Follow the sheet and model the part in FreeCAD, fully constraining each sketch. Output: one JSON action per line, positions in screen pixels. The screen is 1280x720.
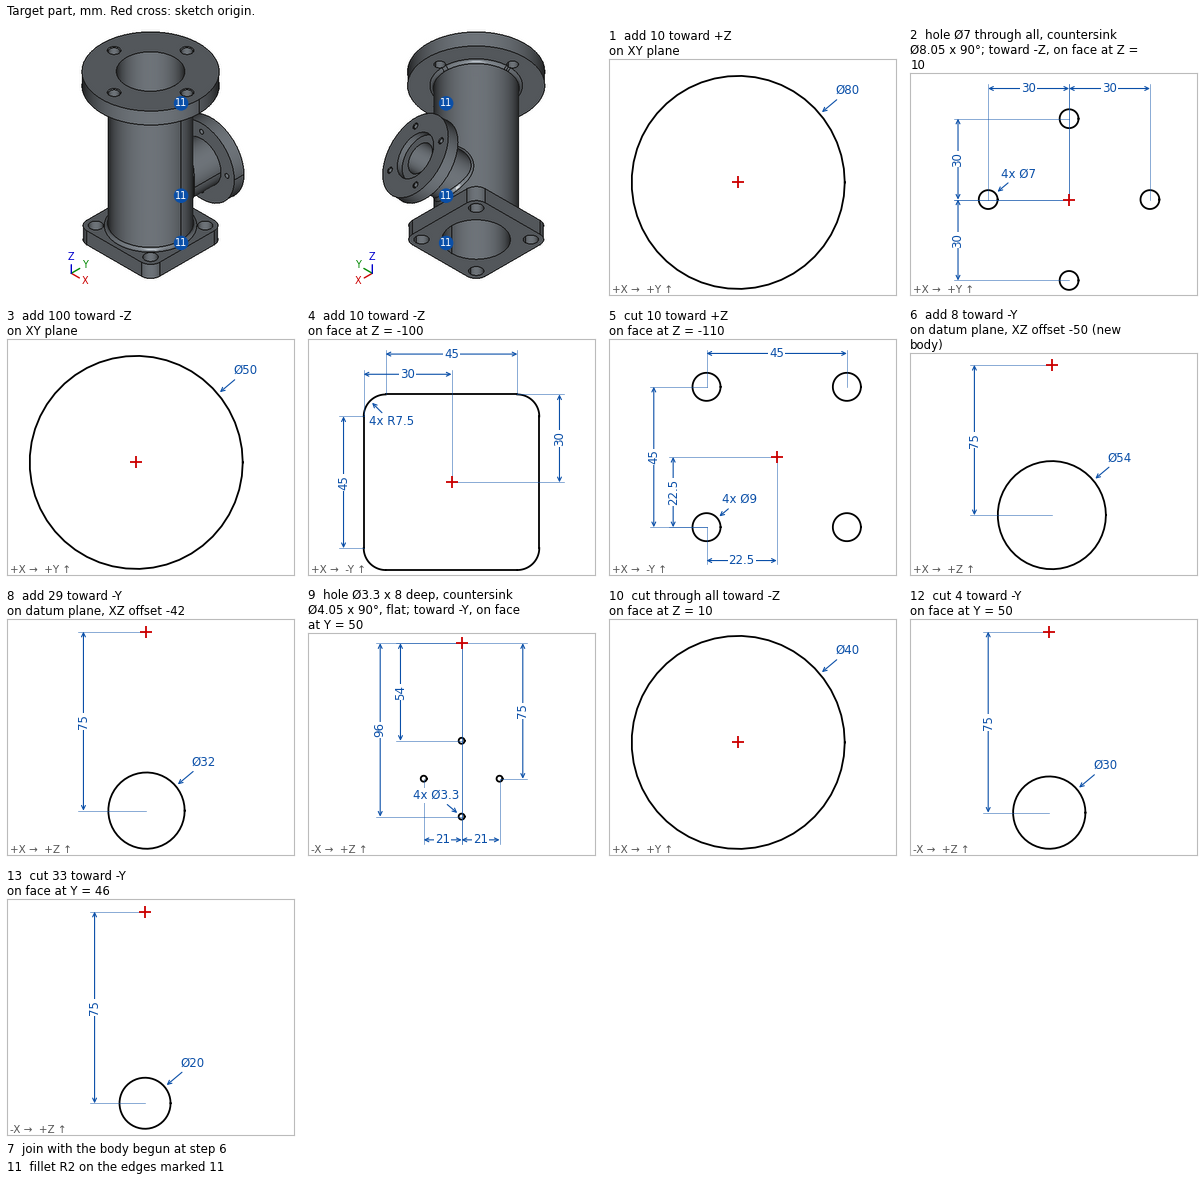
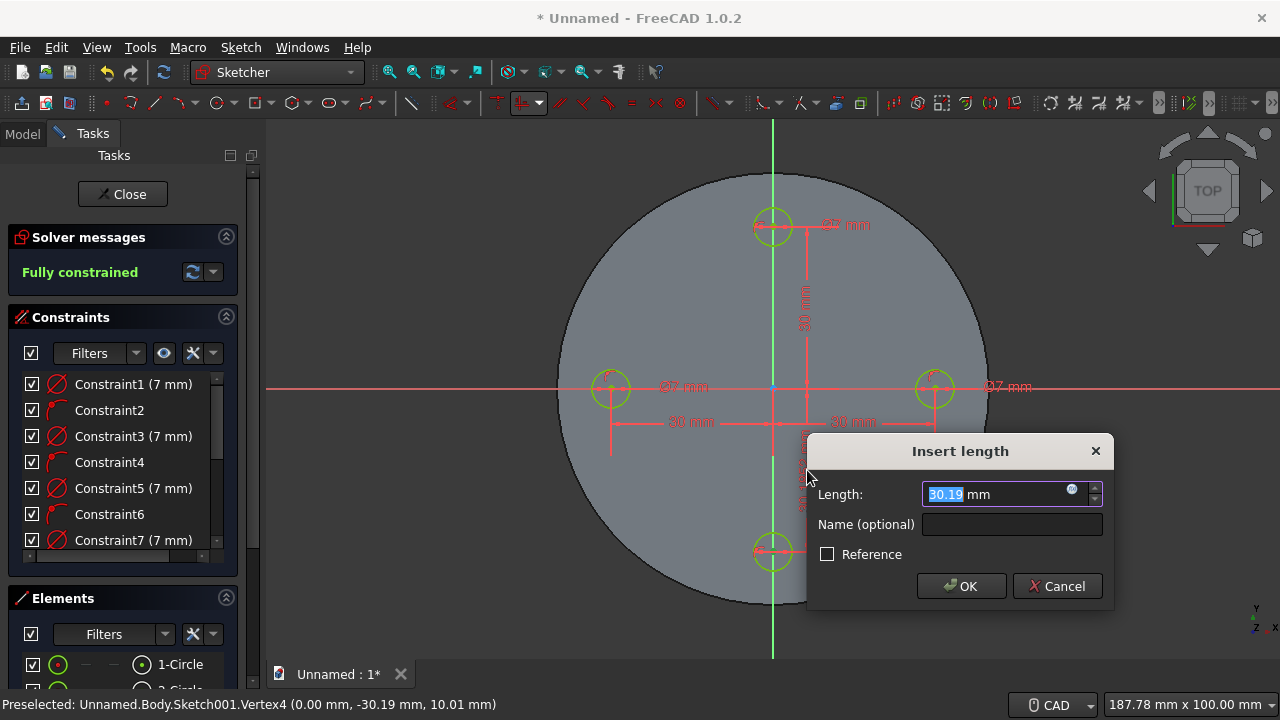
{"action": "type", "text": "30"}
{"action": "key", "text": "Return"}
{"action": "key", "text": "Escape"}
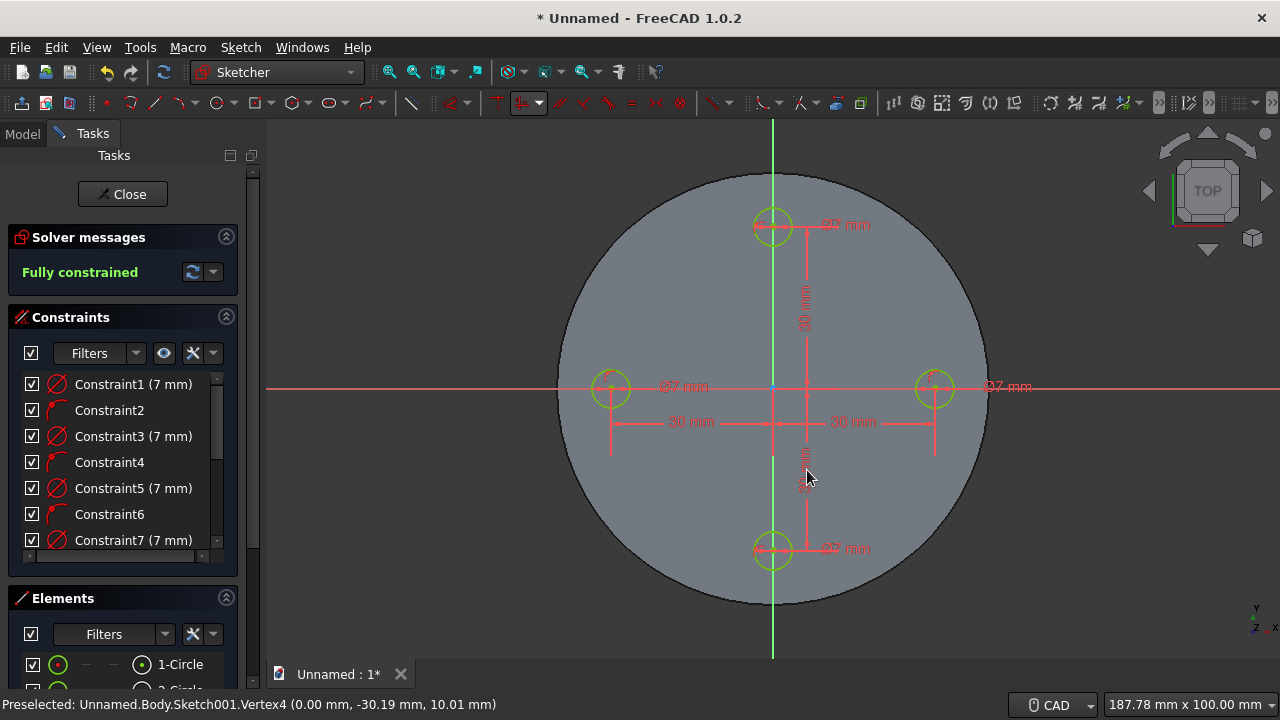
{"action": "left_click", "coordinate": [123, 194]}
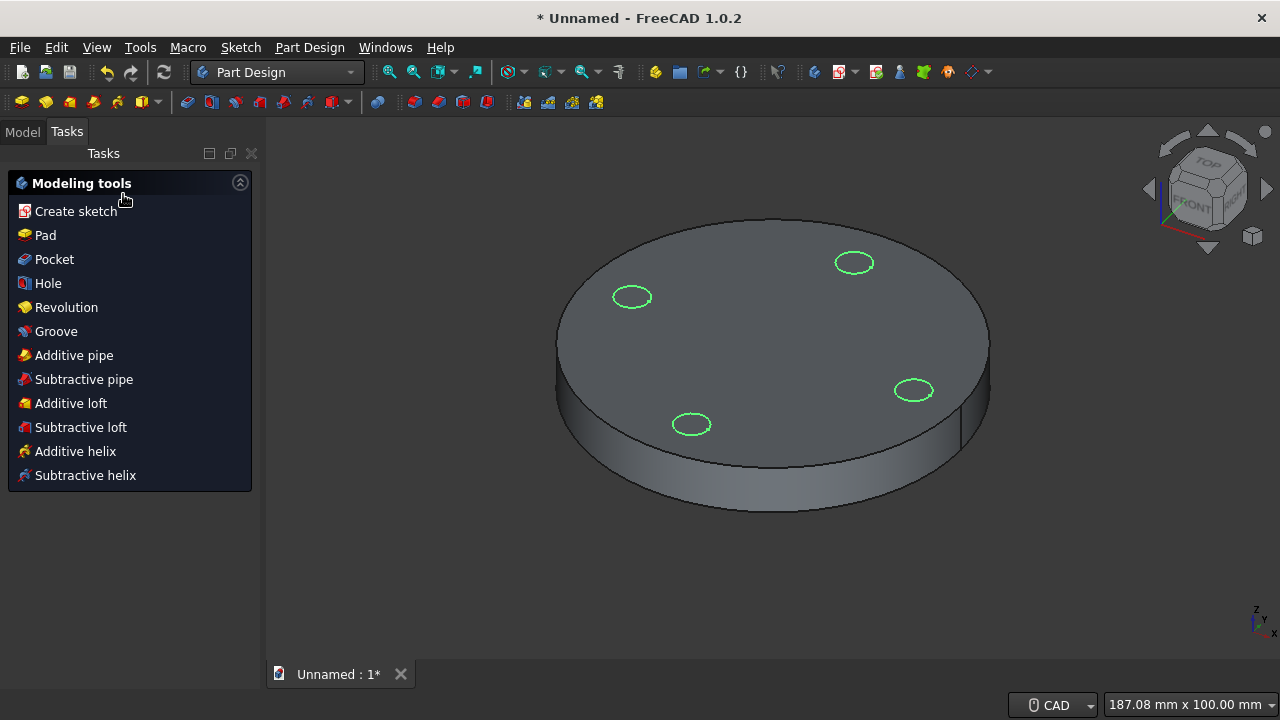
{"action": "left_click", "coordinate": [212, 102]}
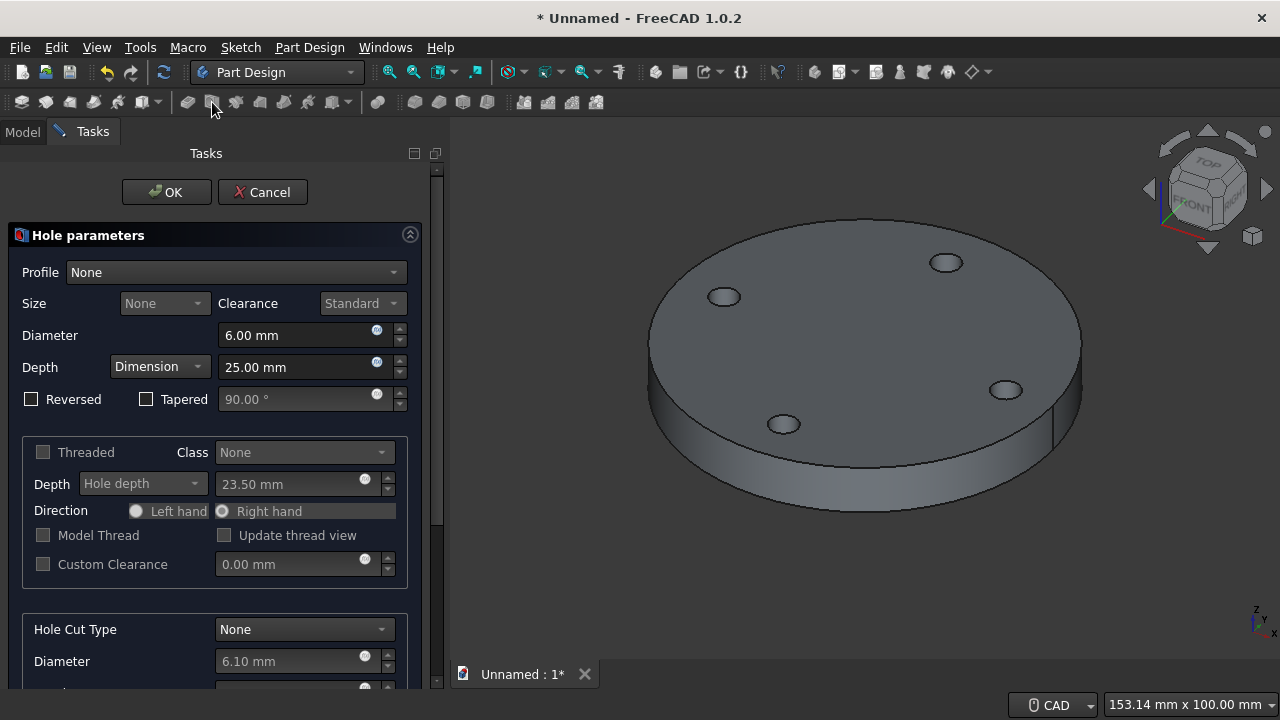
{"action": "triple_click", "coordinate": [305, 335]}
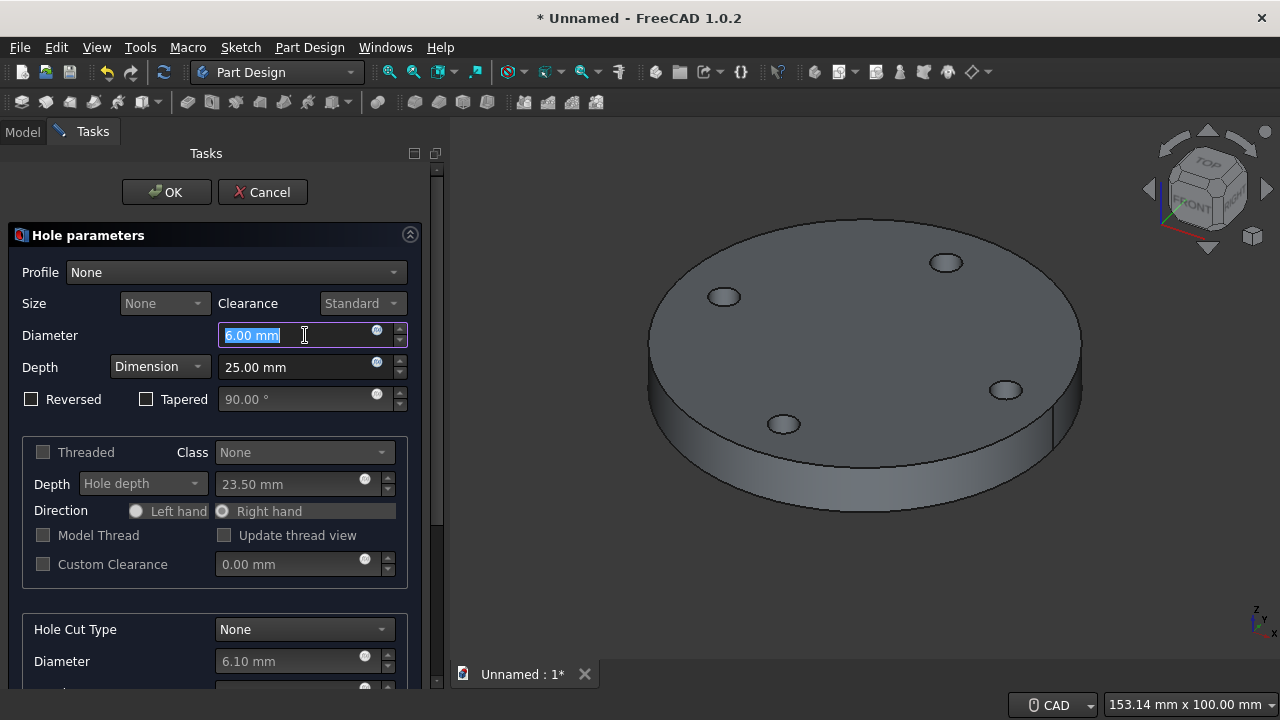
{"action": "type", "text": "7"}
{"action": "key", "text": "Tab"}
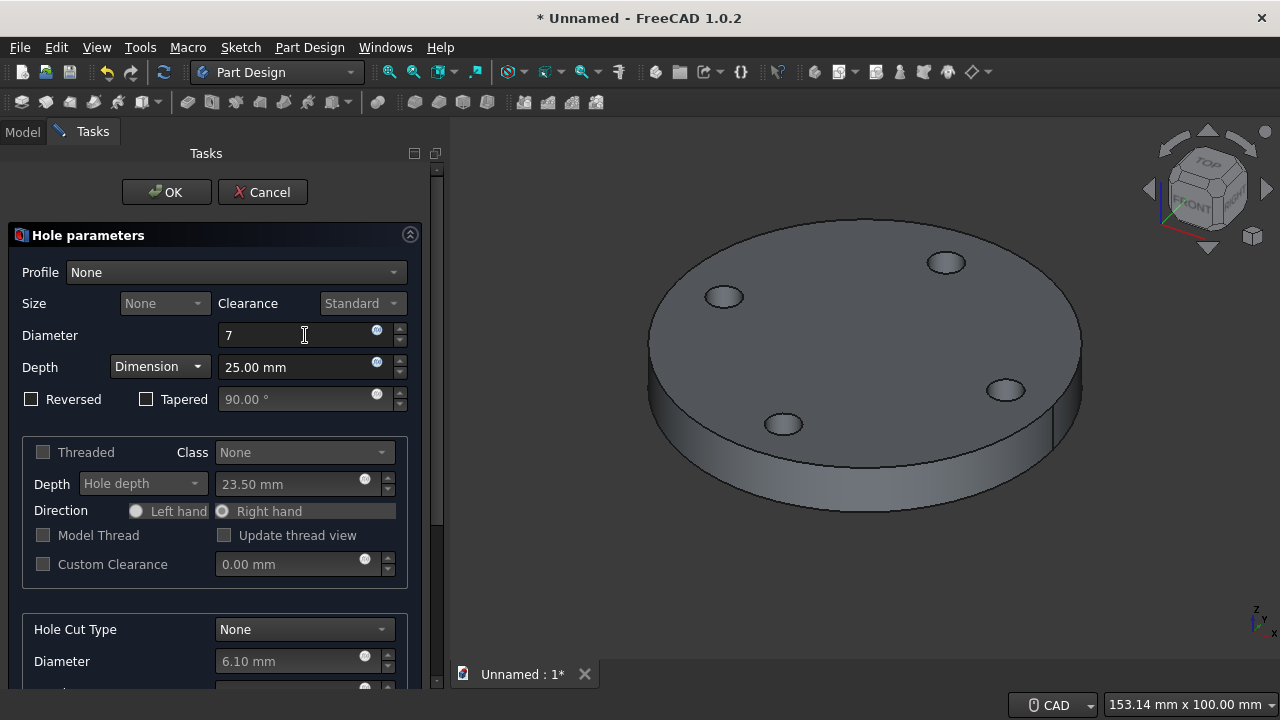
{"action": "left_click", "coordinate": [161, 366]}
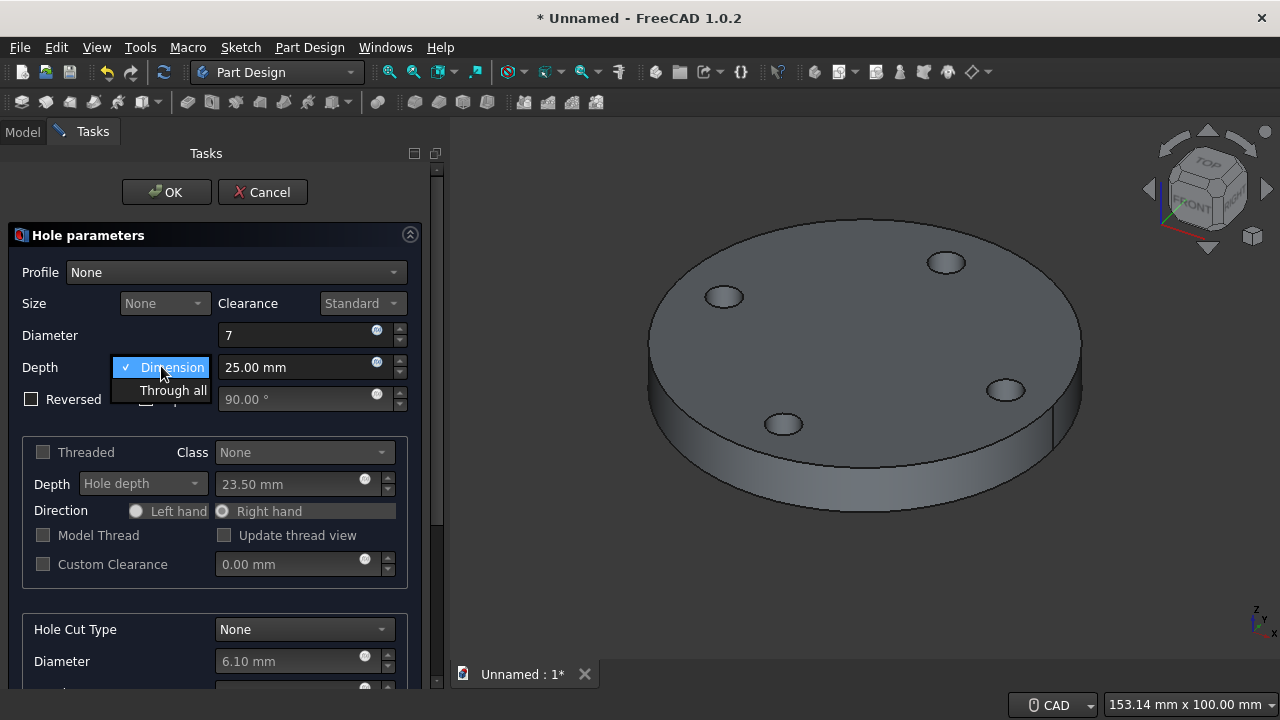
{"action": "left_click", "coordinate": [160, 390]}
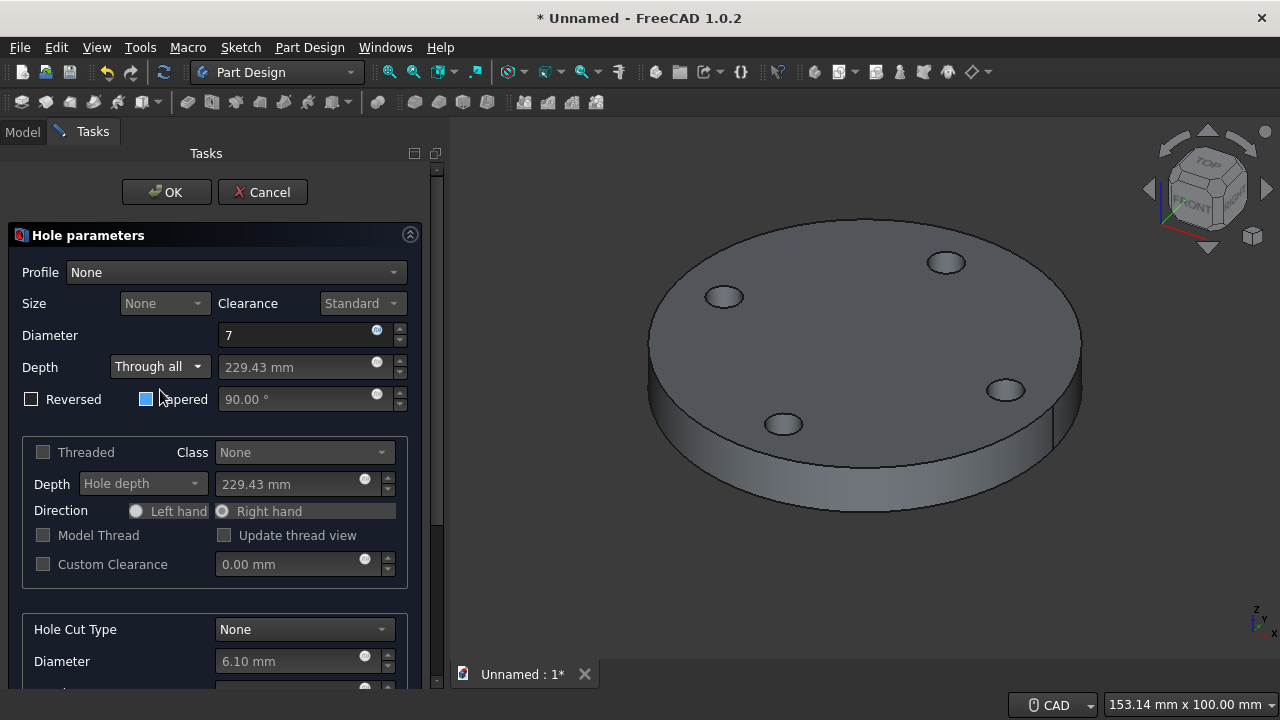
{"action": "left_click", "coordinate": [306, 630]}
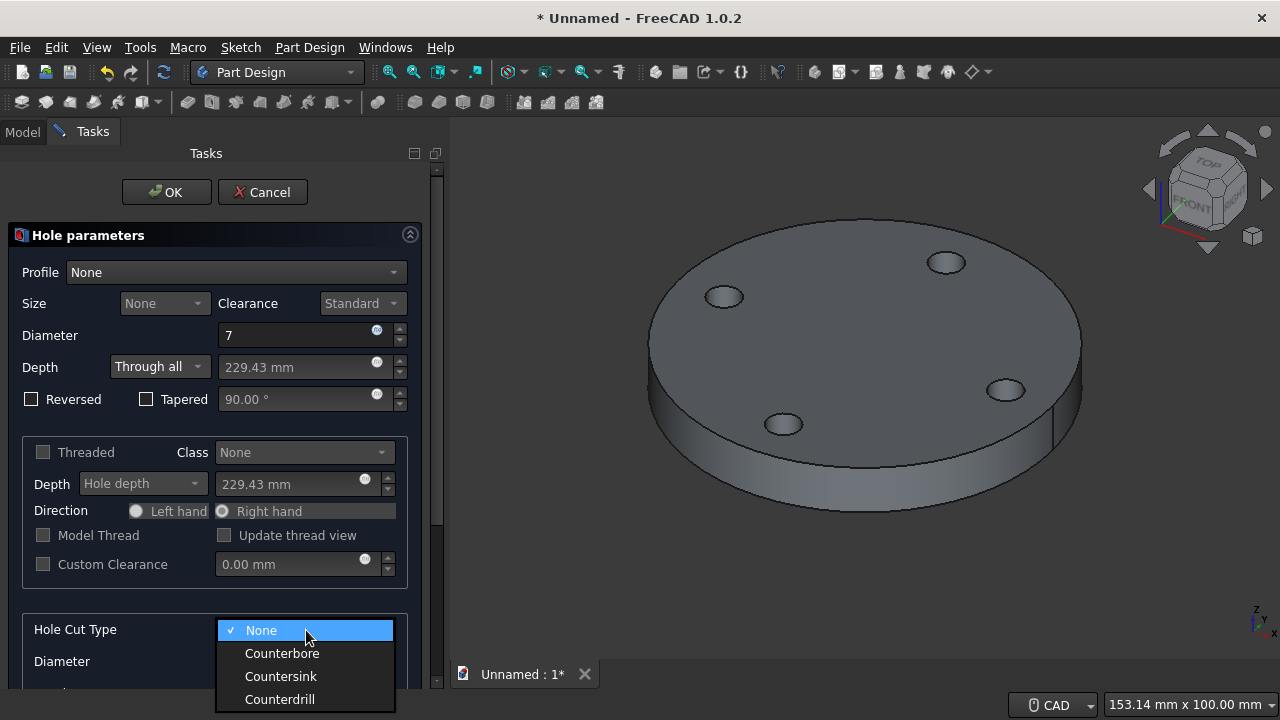
{"action": "left_click", "coordinate": [304, 676]}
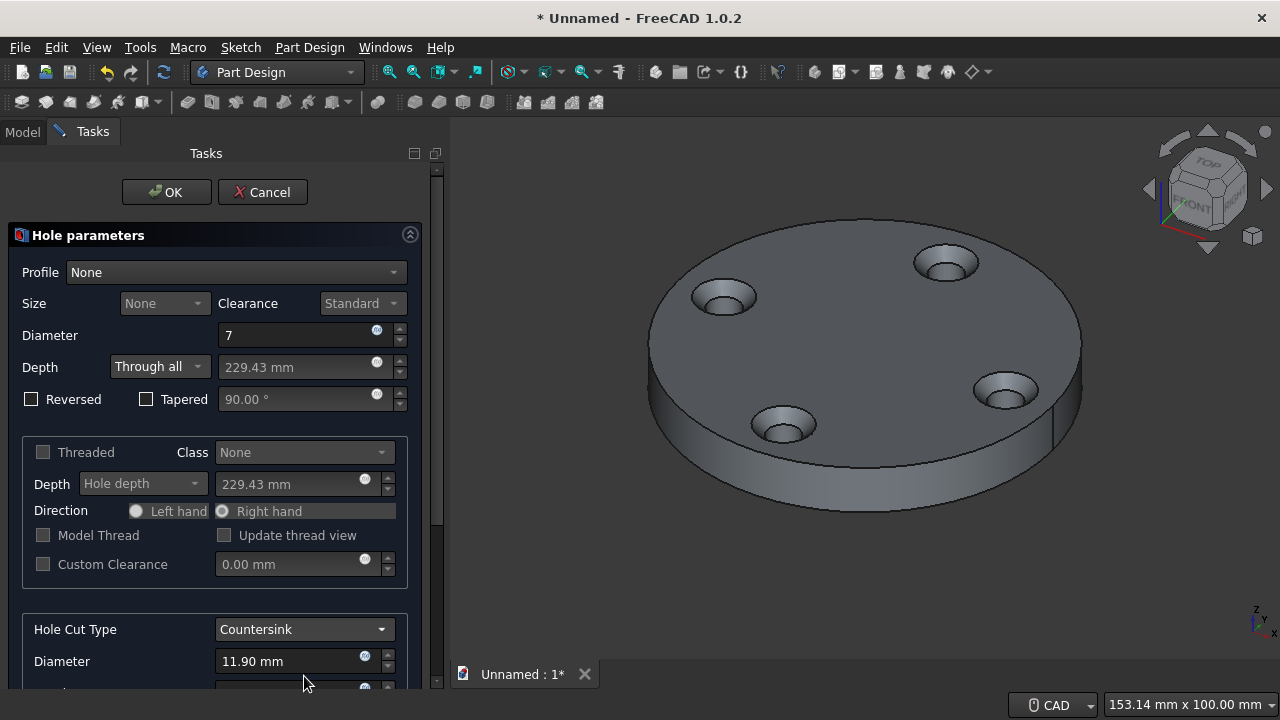
{"action": "triple_click", "coordinate": [298, 661]}